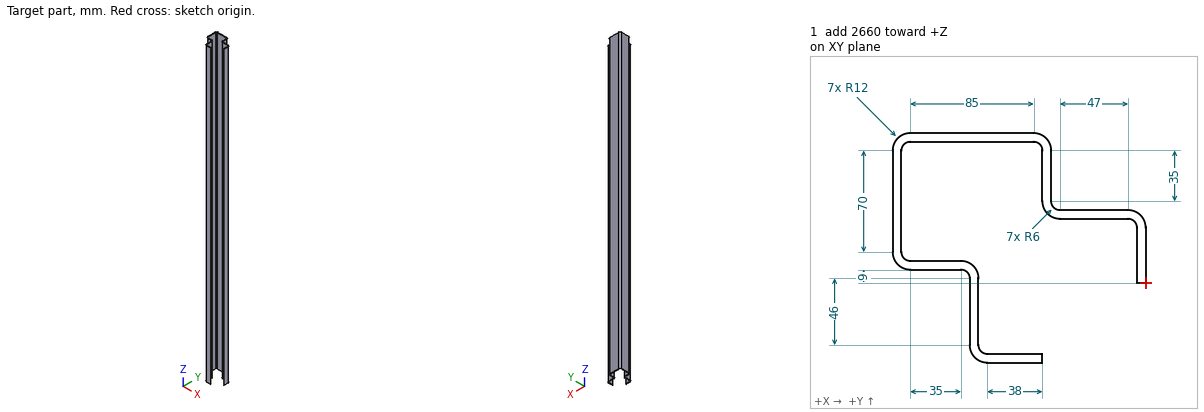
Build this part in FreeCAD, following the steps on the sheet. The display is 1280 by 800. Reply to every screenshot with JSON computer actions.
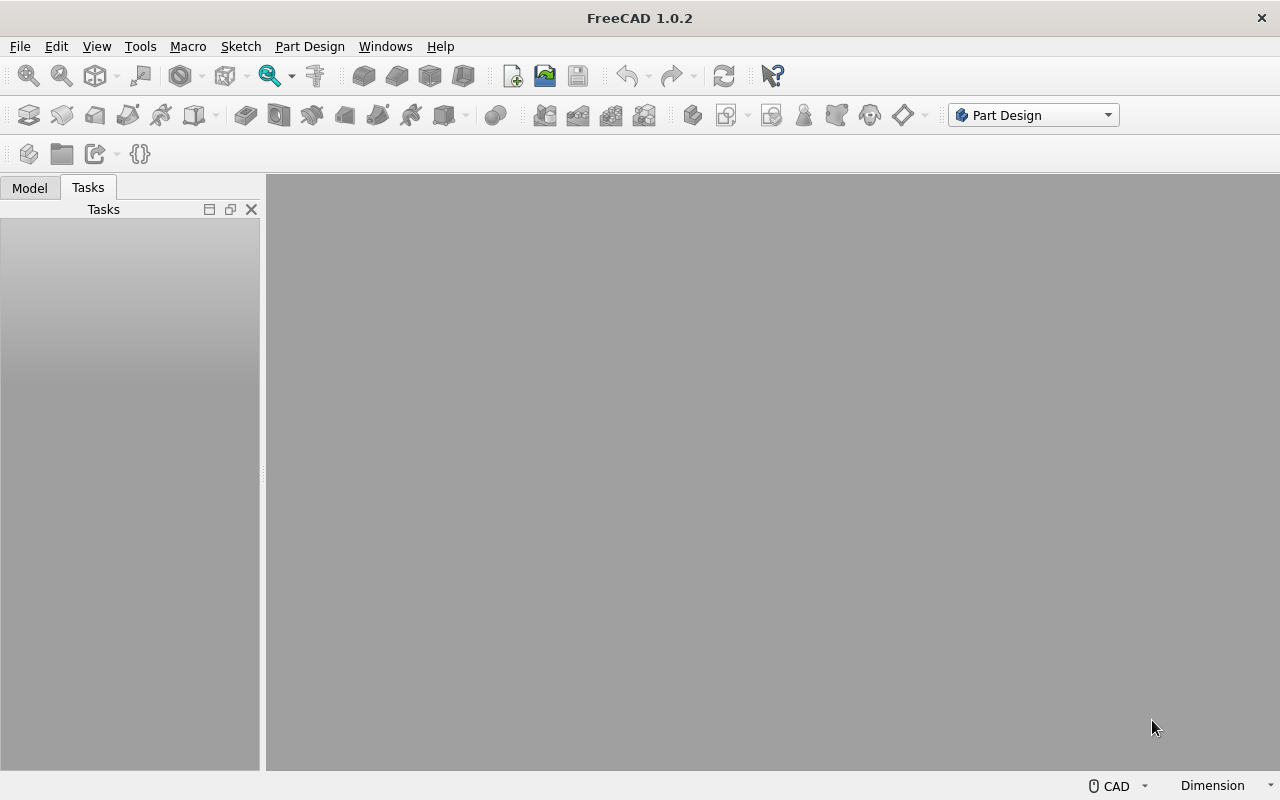
{"action": "key", "text": "ctrl+n"}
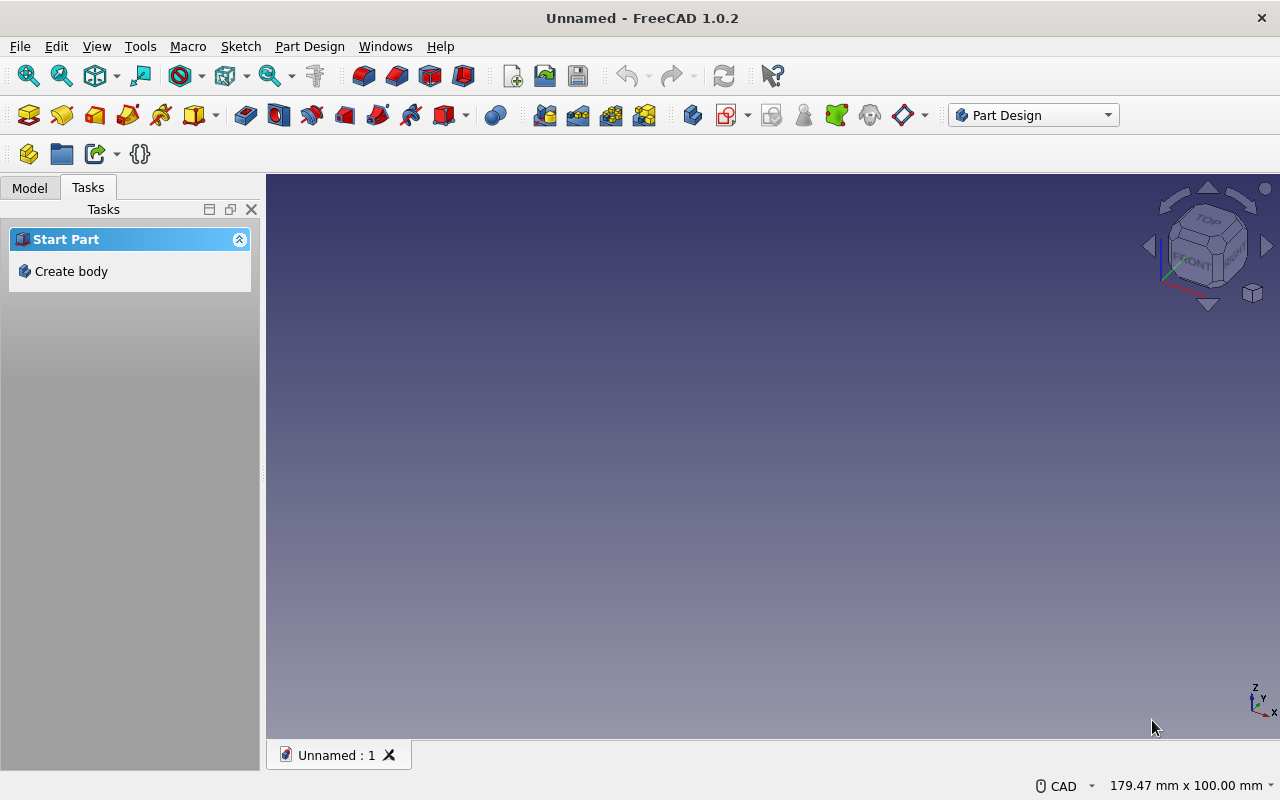
{"action": "left_click", "coordinate": [726, 116]}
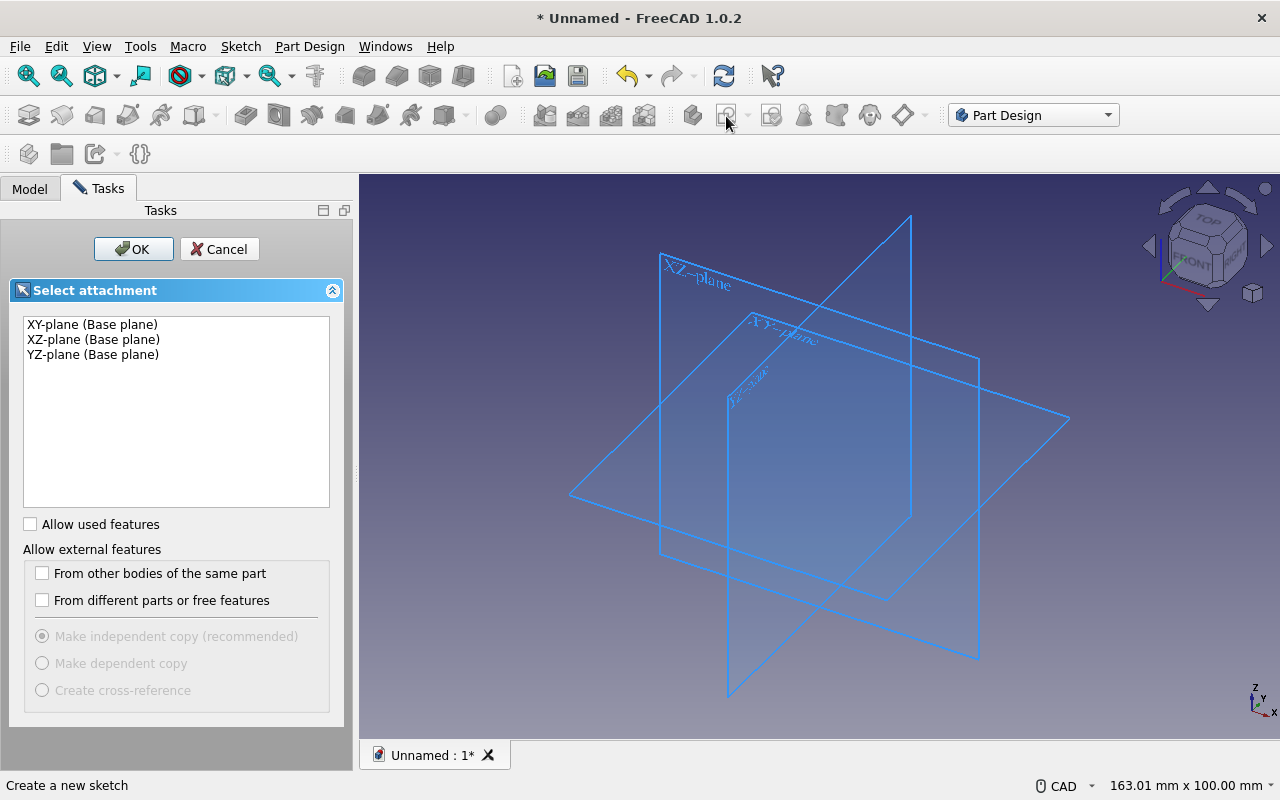
{"action": "left_click", "coordinate": [84, 324]}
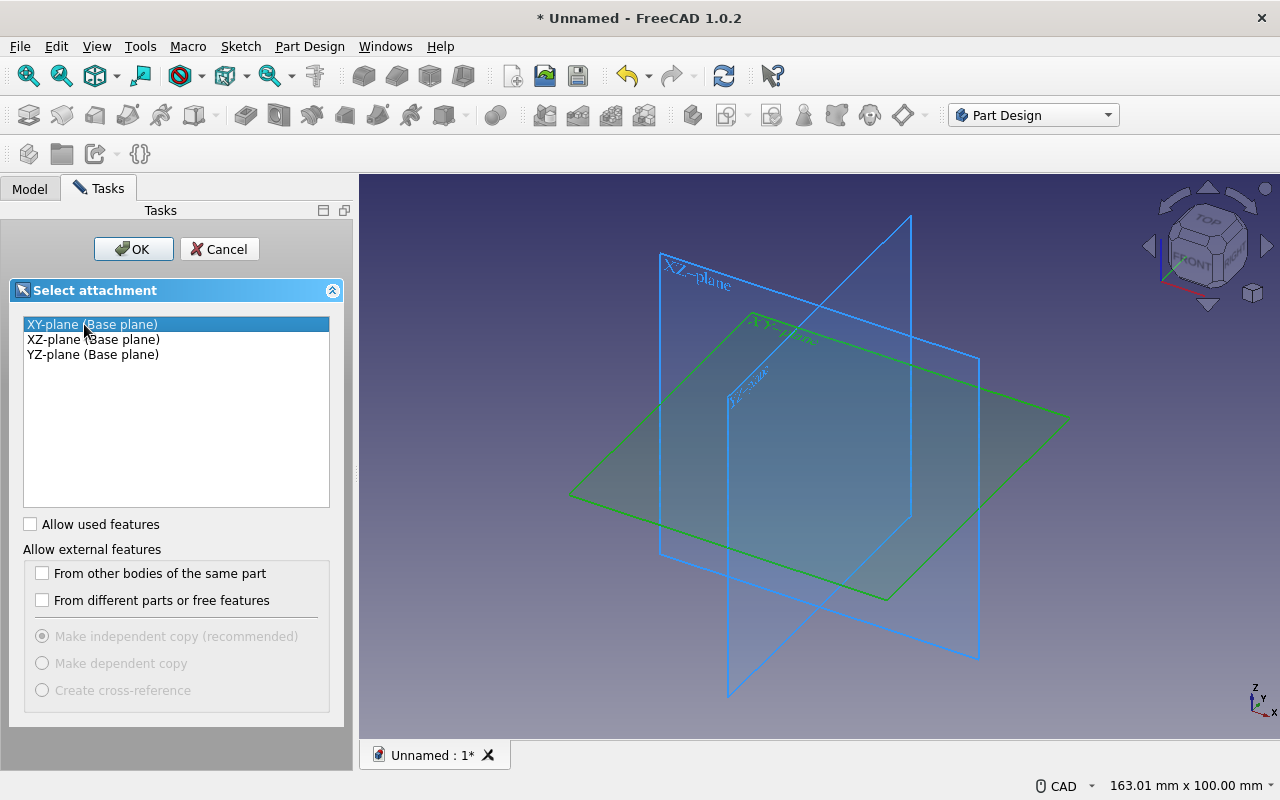
{"action": "left_click", "coordinate": [134, 249]}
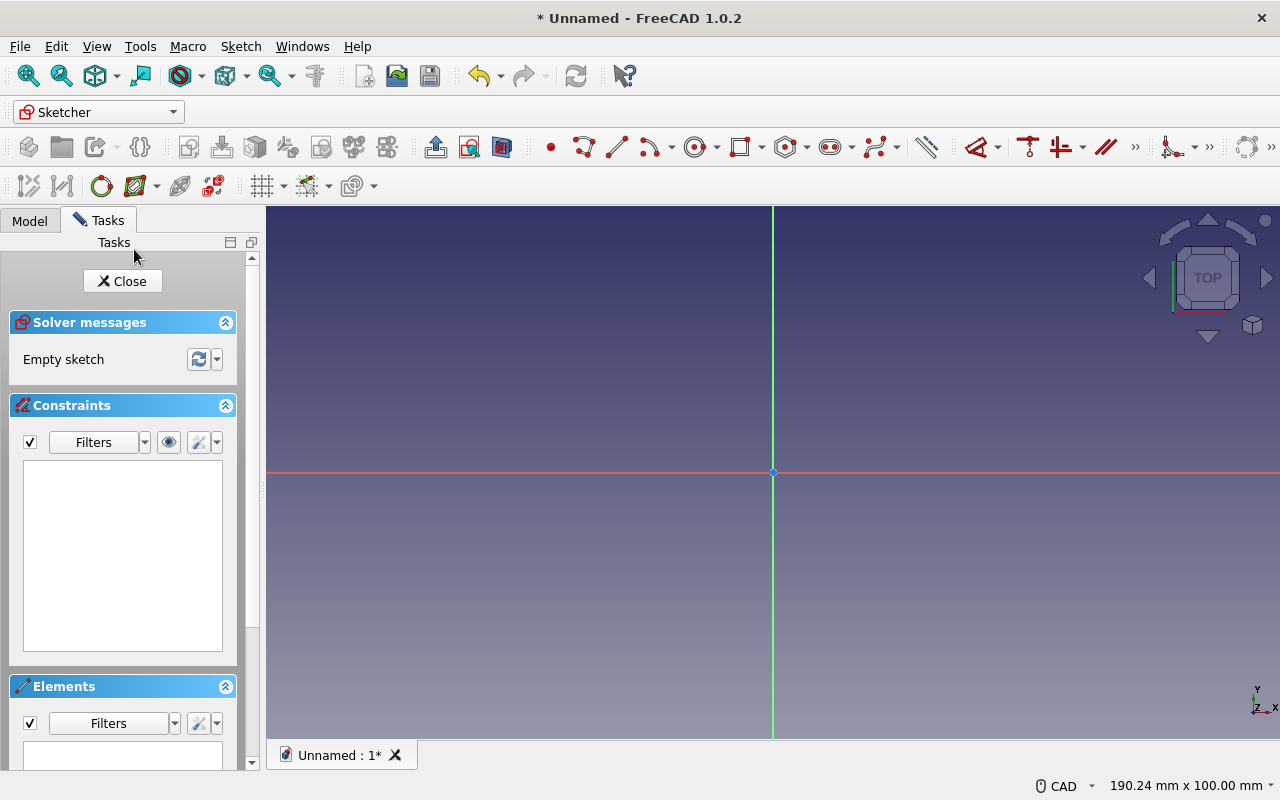
{"action": "scroll", "coordinate": [935, 547], "scroll_direction": "down", "scroll_amount": 5}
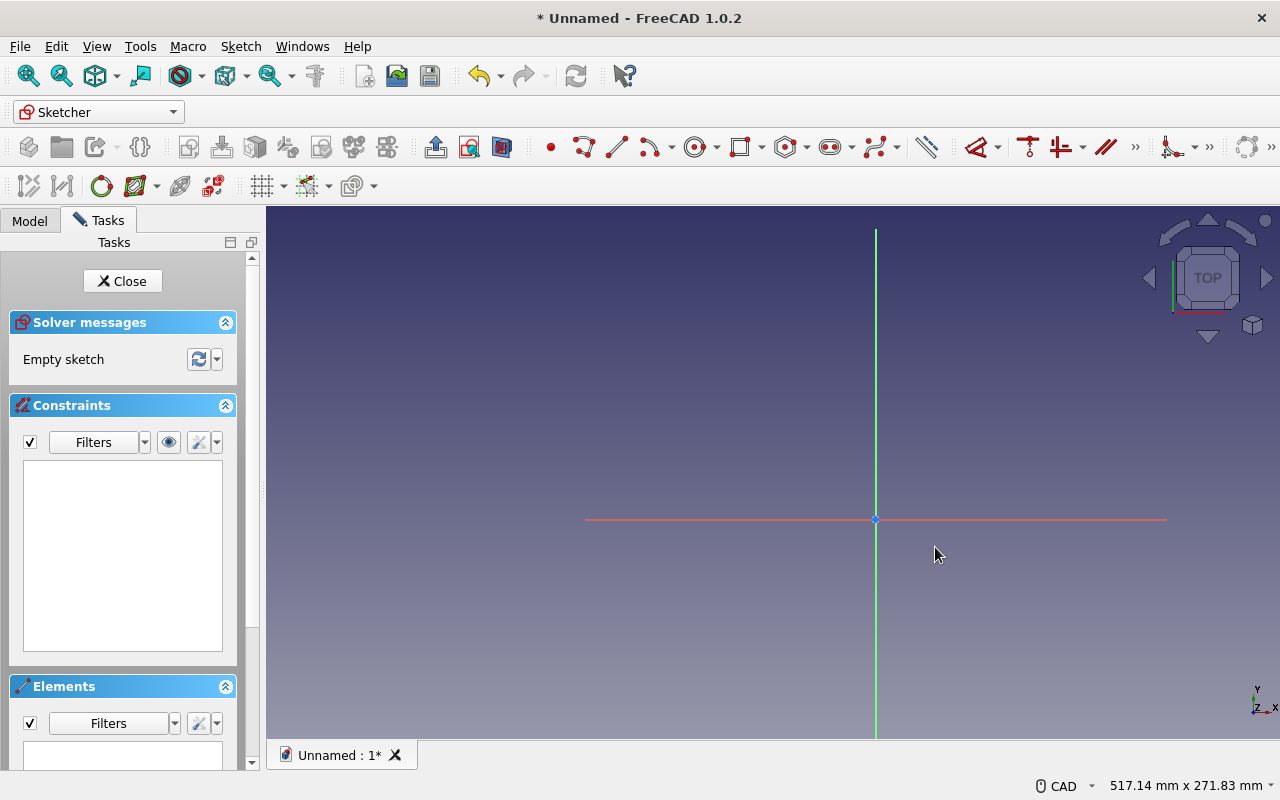
{"action": "key", "text": "g l"}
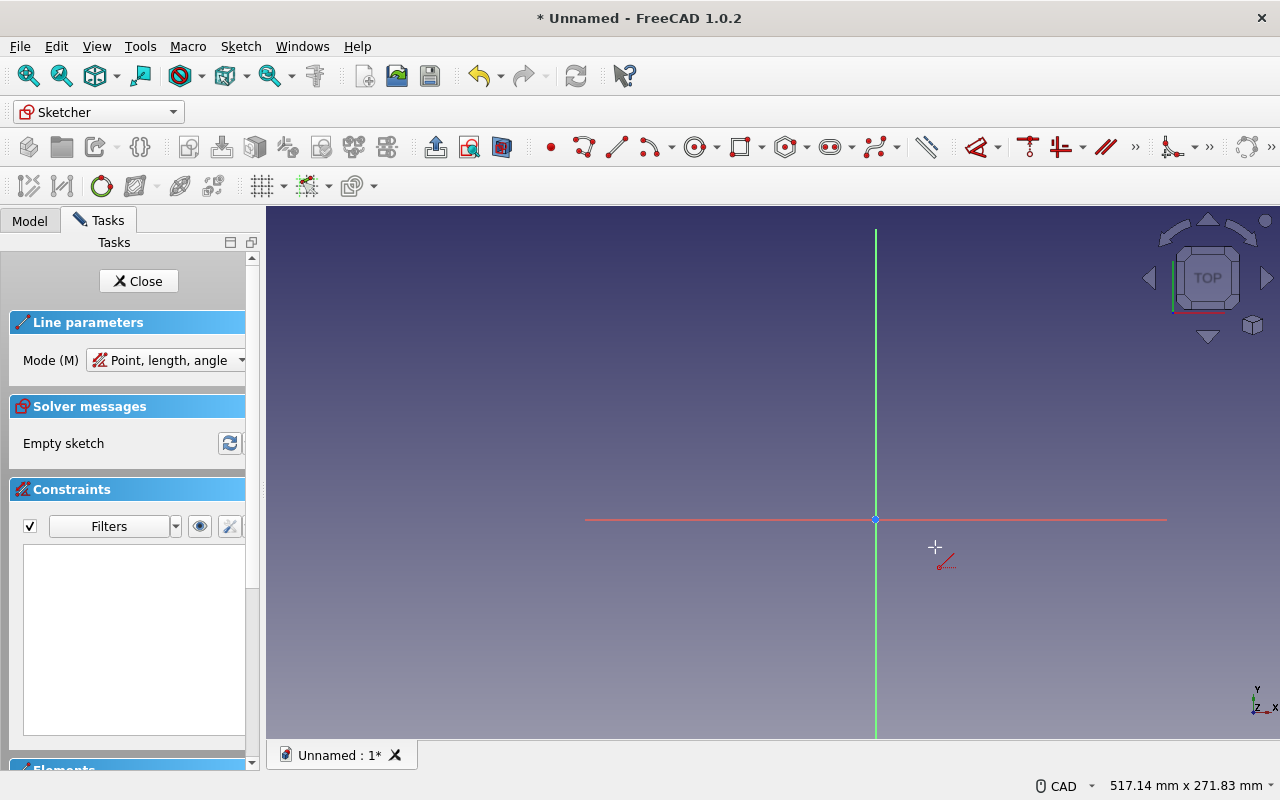
{"action": "left_click", "coordinate": [852, 422]}
{"action": "left_click", "coordinate": [760, 422]}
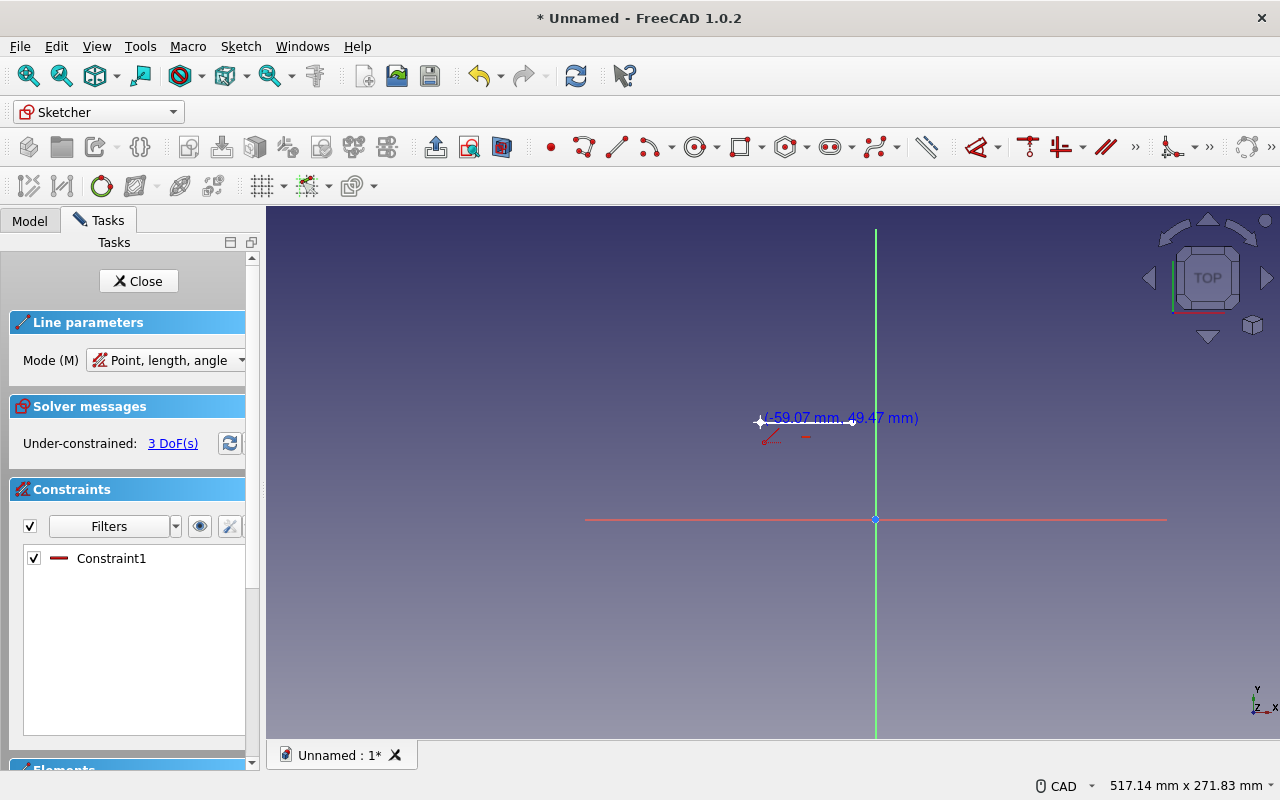
{"action": "left_click", "coordinate": [748, 410]}
{"action": "left_click", "coordinate": [748, 342]}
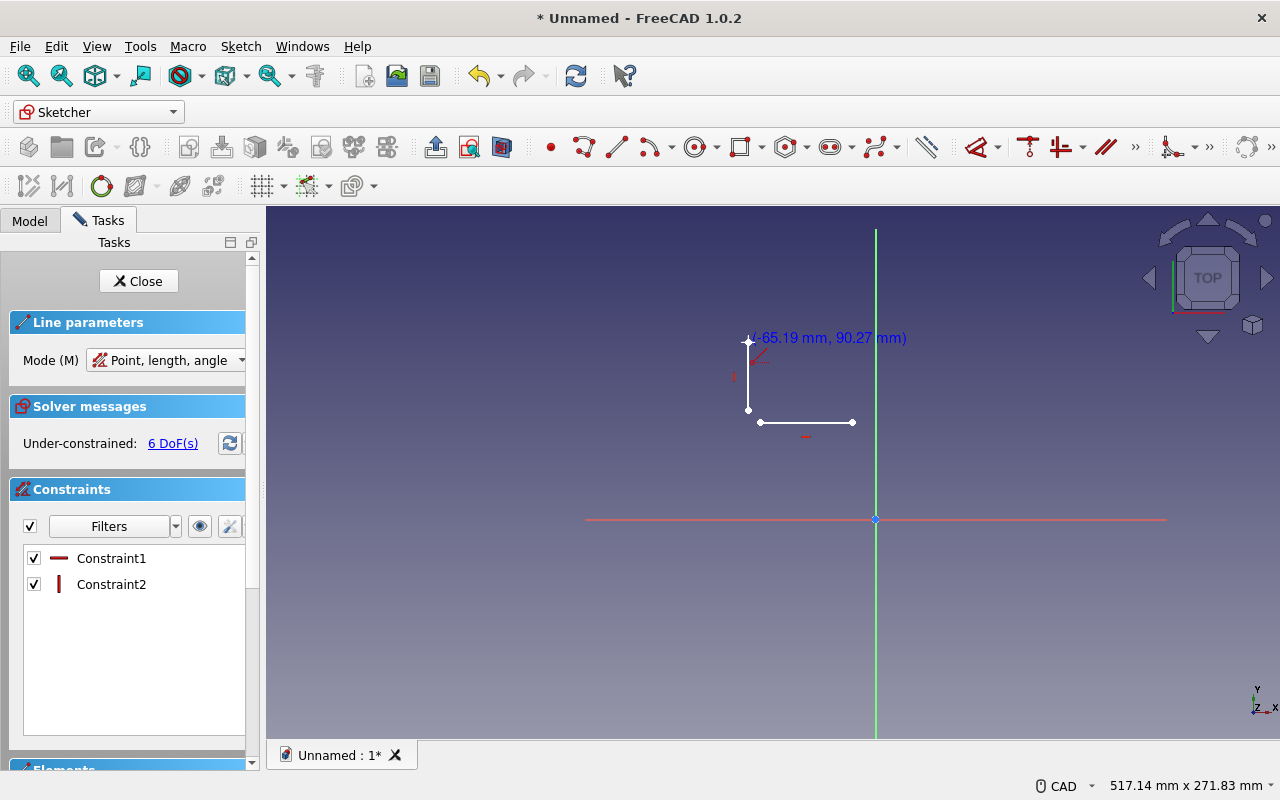
{"action": "left_click", "coordinate": [725, 318]}
{"action": "left_click", "coordinate": [558, 318]}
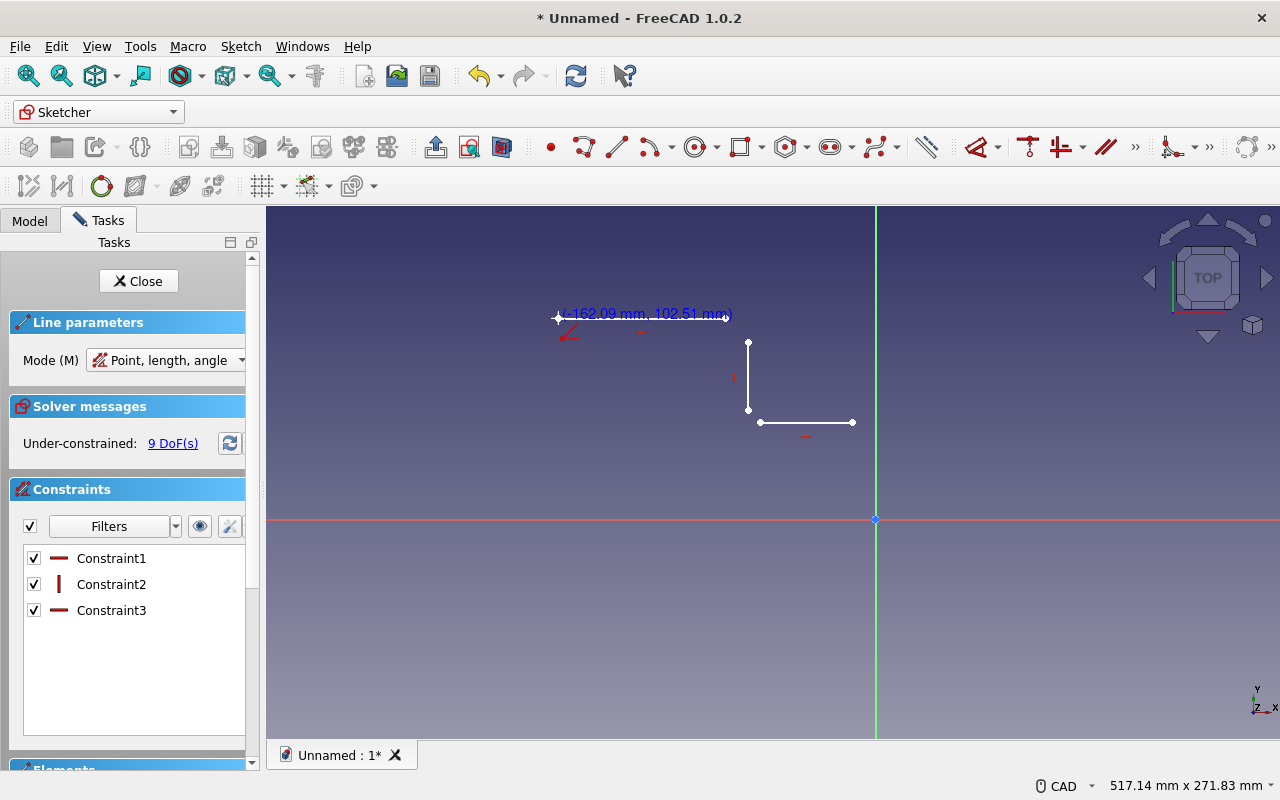
{"action": "left_click", "coordinate": [535, 342]}
{"action": "left_click", "coordinate": [535, 479]}